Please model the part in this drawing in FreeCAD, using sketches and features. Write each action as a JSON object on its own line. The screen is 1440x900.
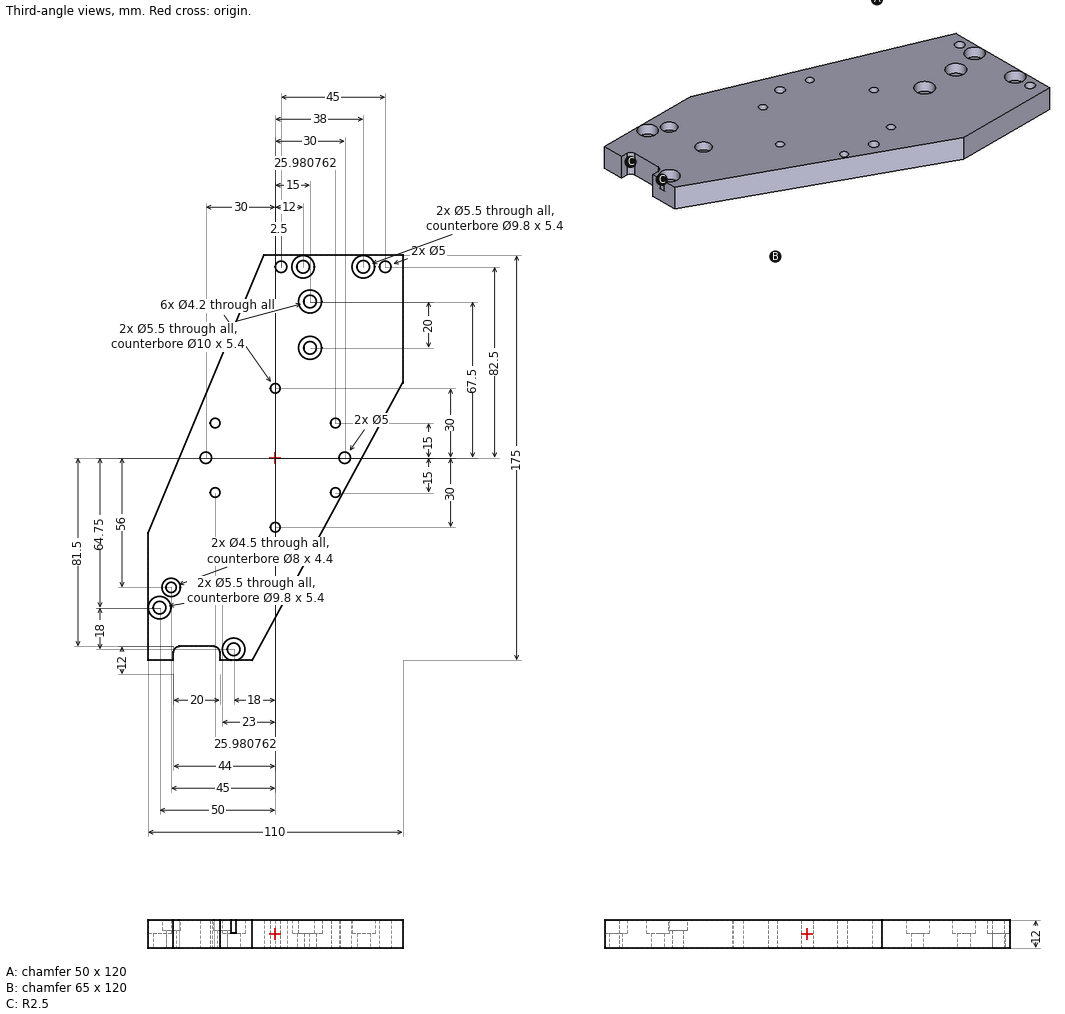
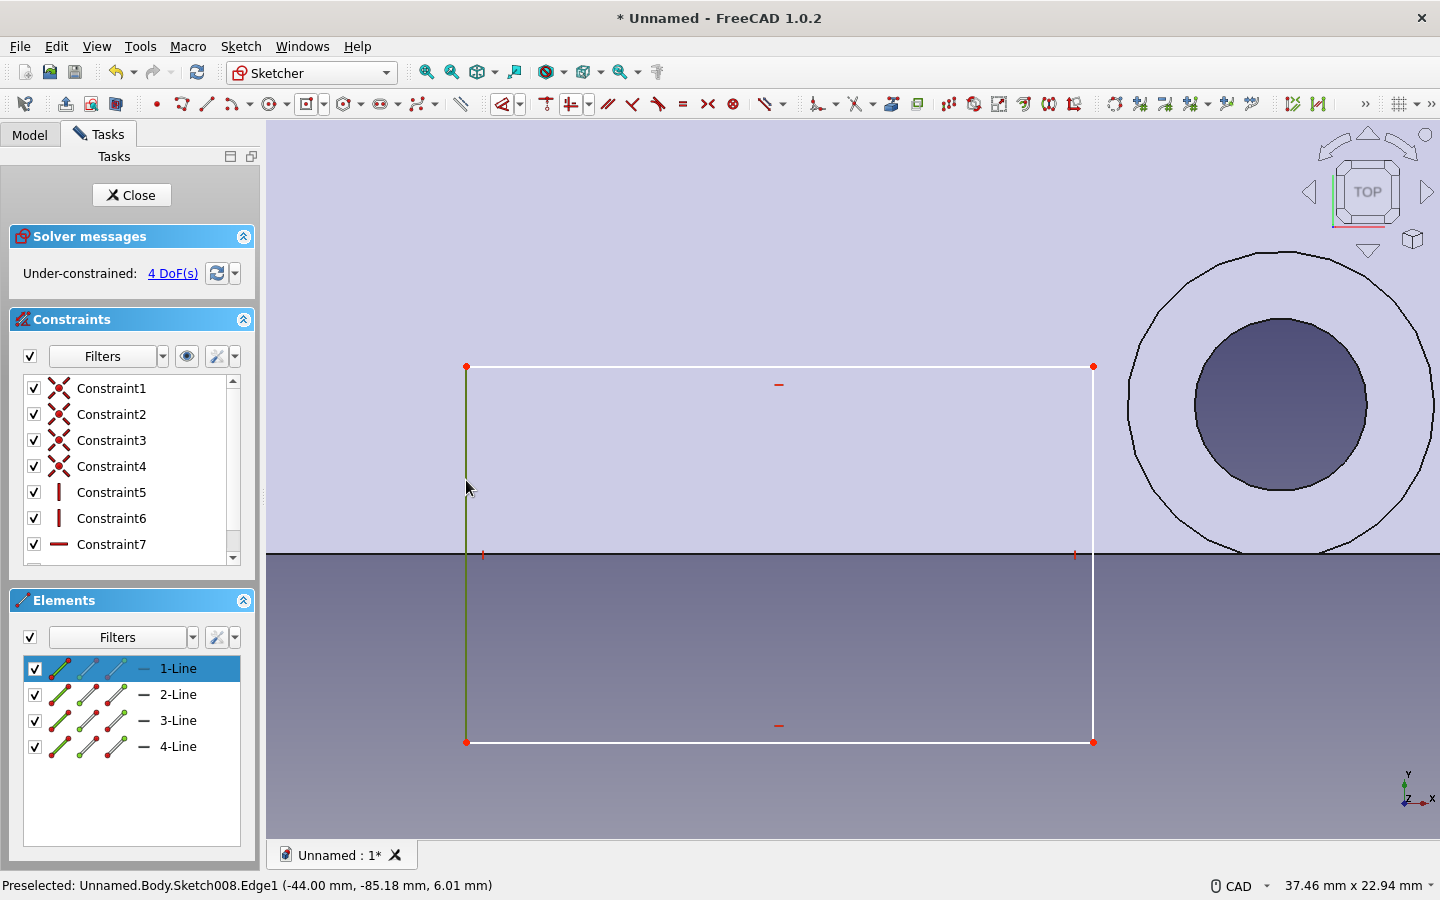
{"action": "key", "text": "i"}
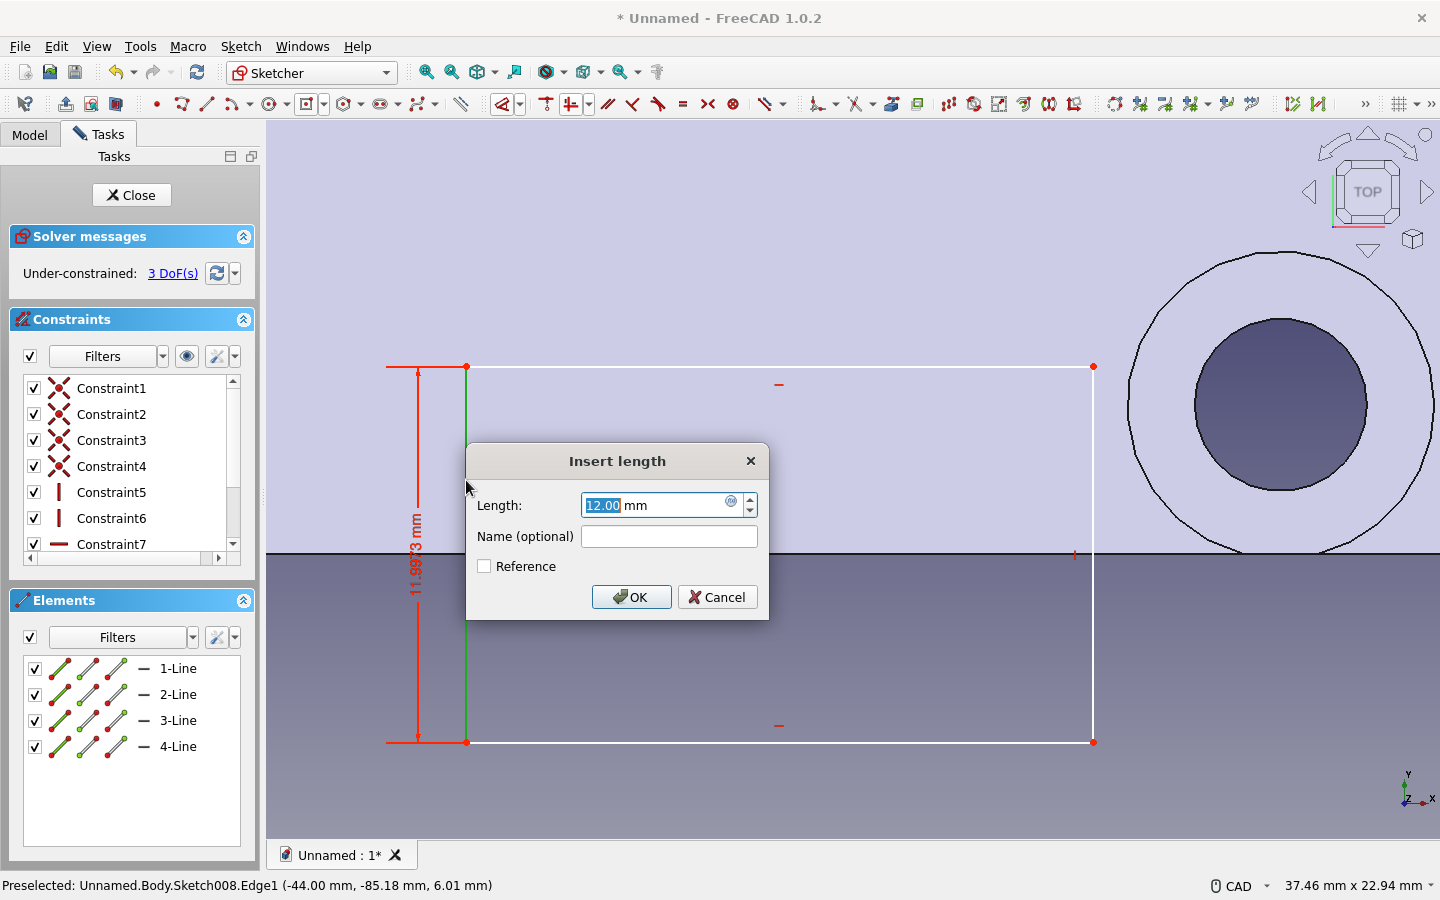
{"action": "type", "text": "12"}
{"action": "key", "text": "Return"}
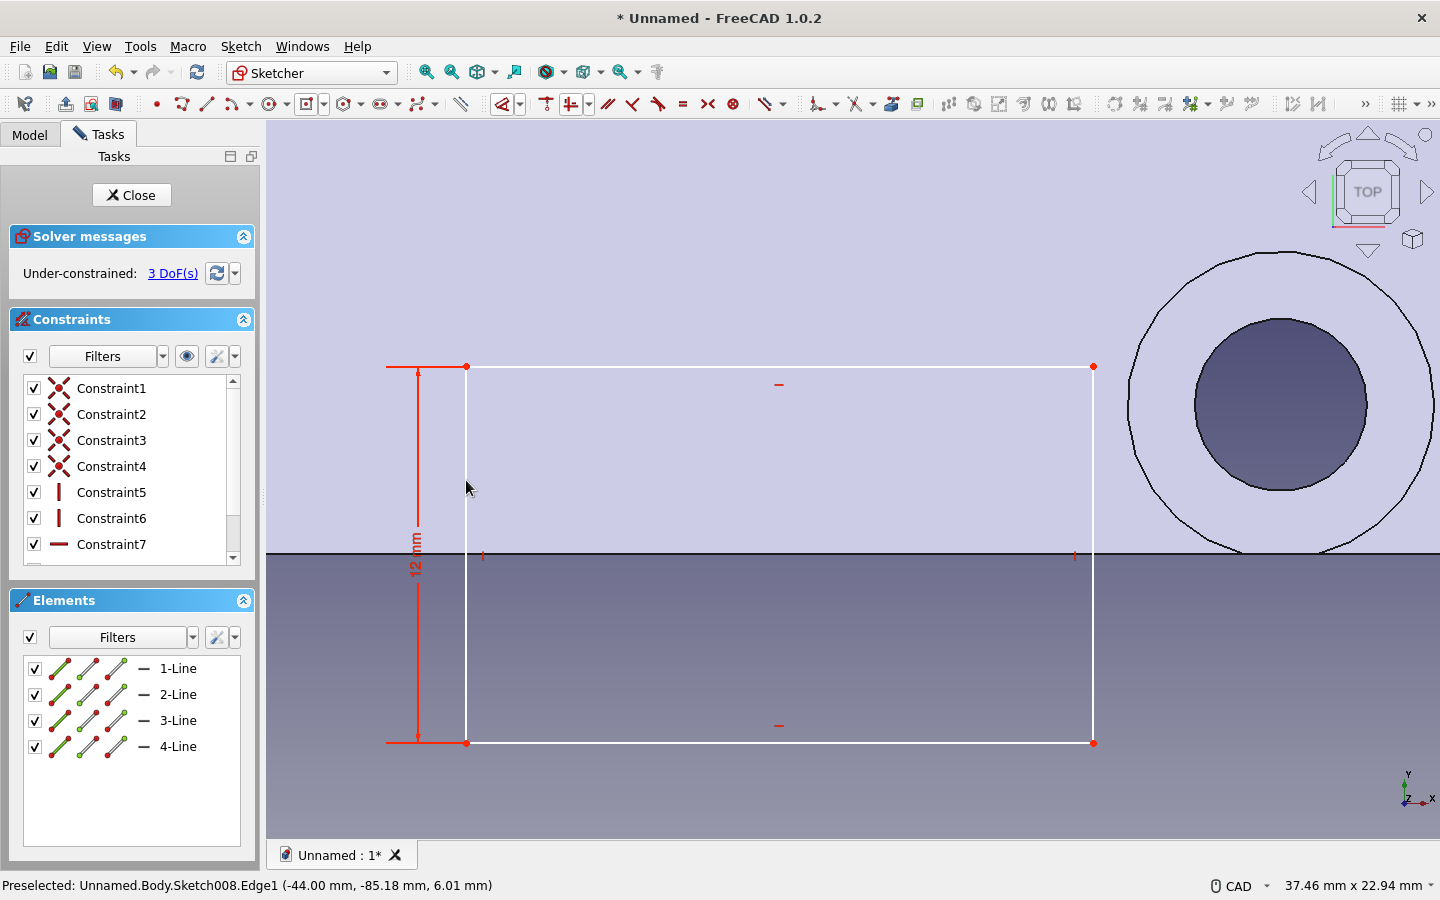
{"action": "left_click", "coordinate": [654, 743]}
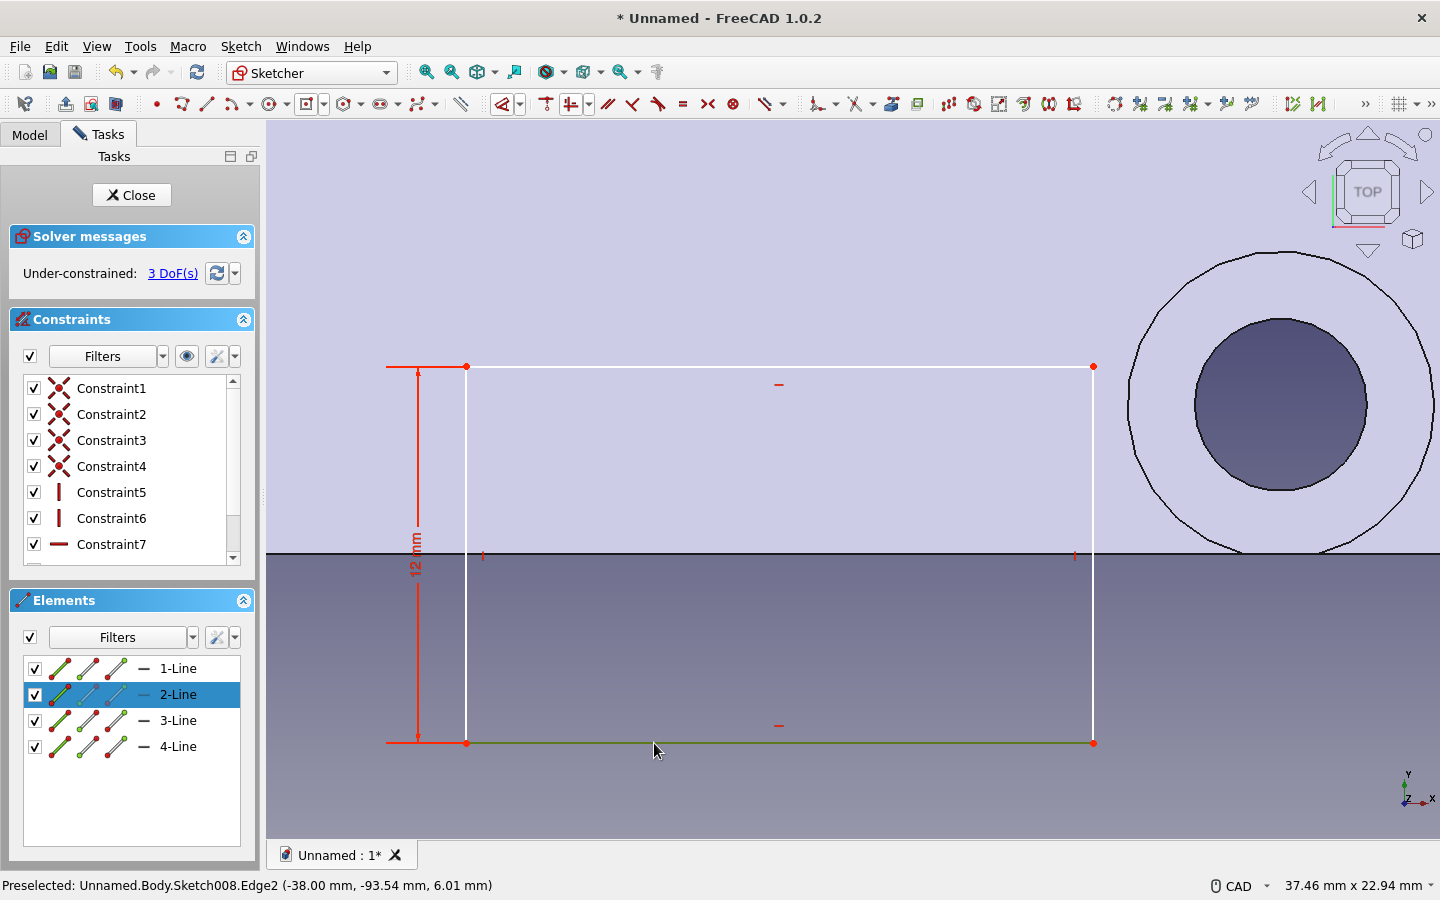
{"action": "key", "text": "l"}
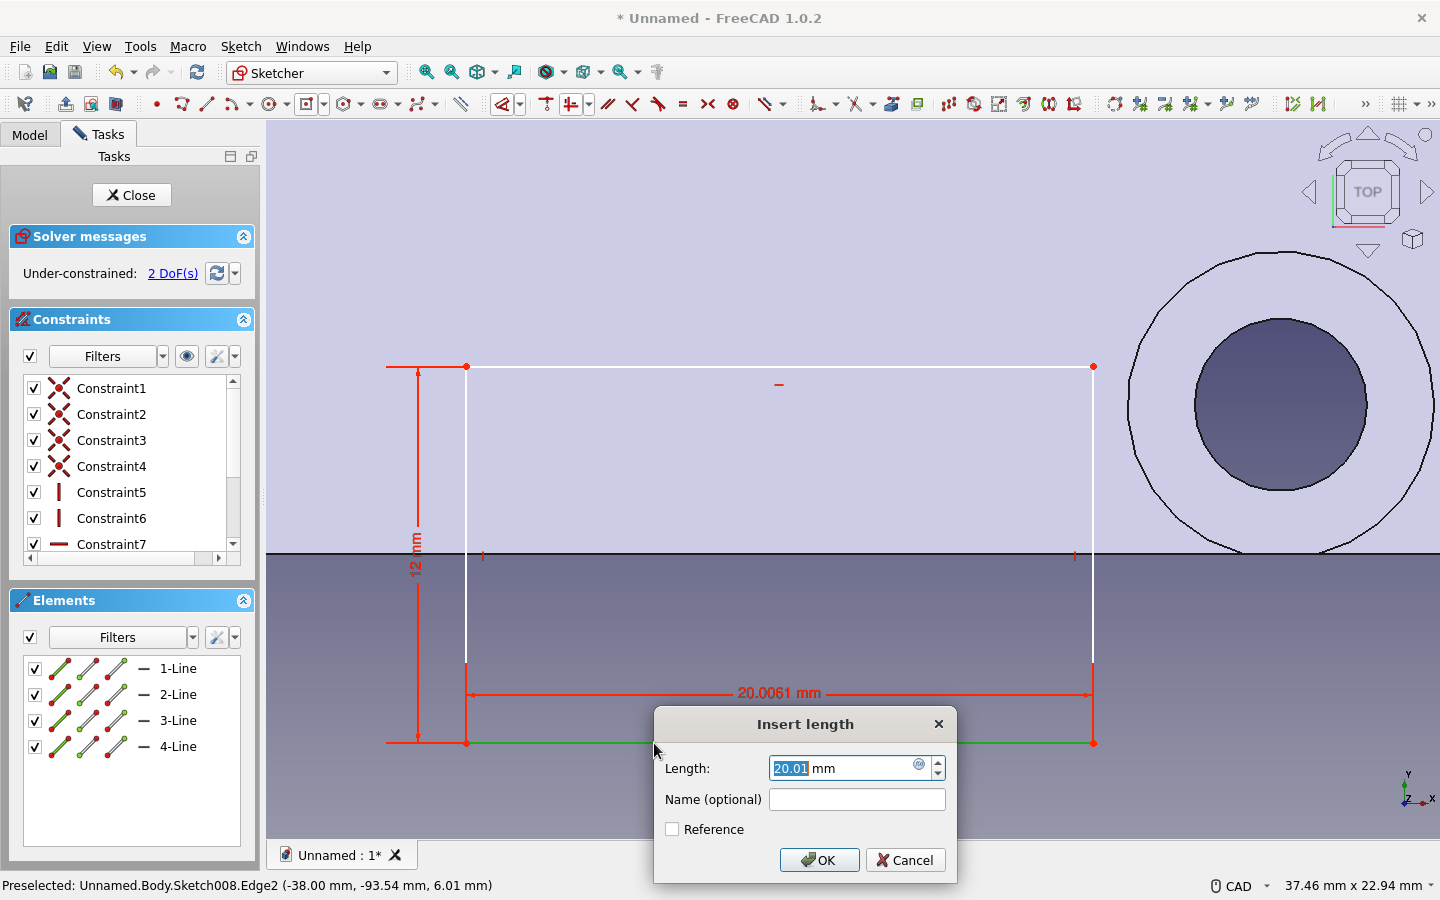
{"action": "type", "text": "20"}
{"action": "key", "text": "Return"}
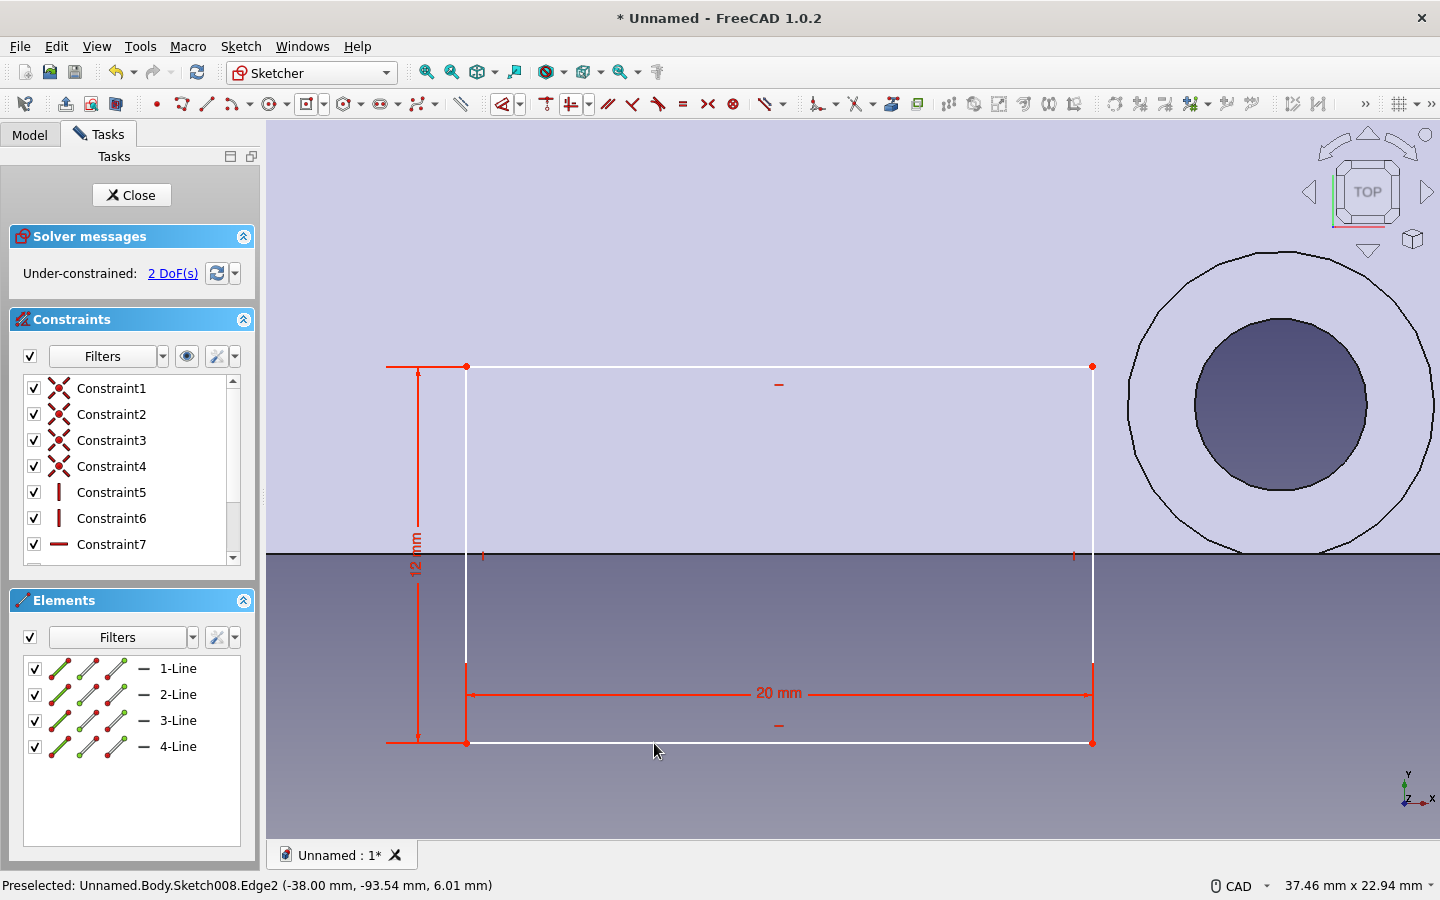
{"action": "left_click", "coordinate": [466, 367]}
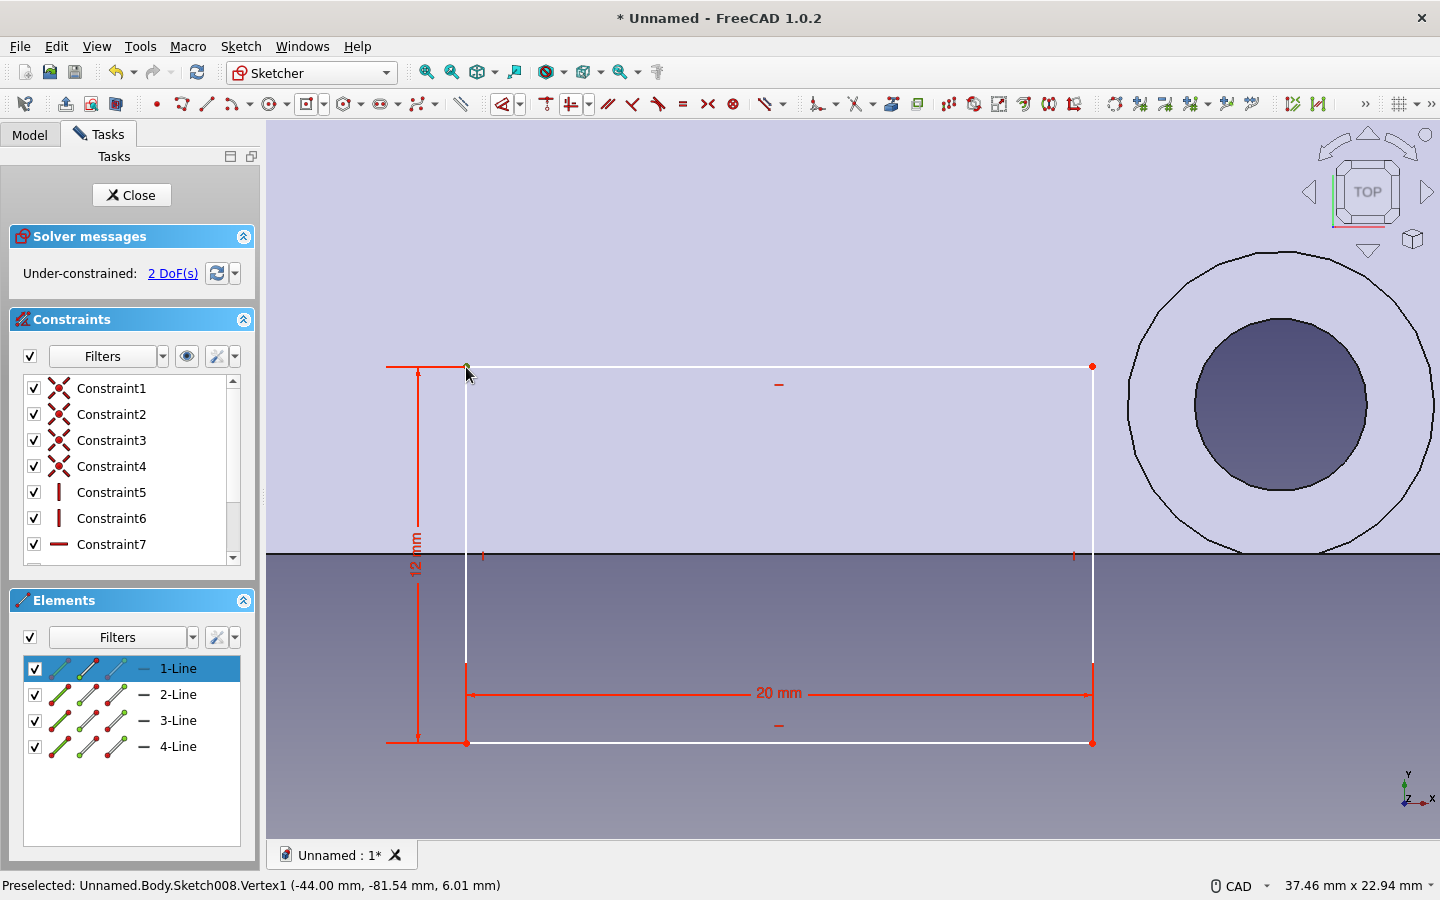
{"action": "key", "text": "l"}